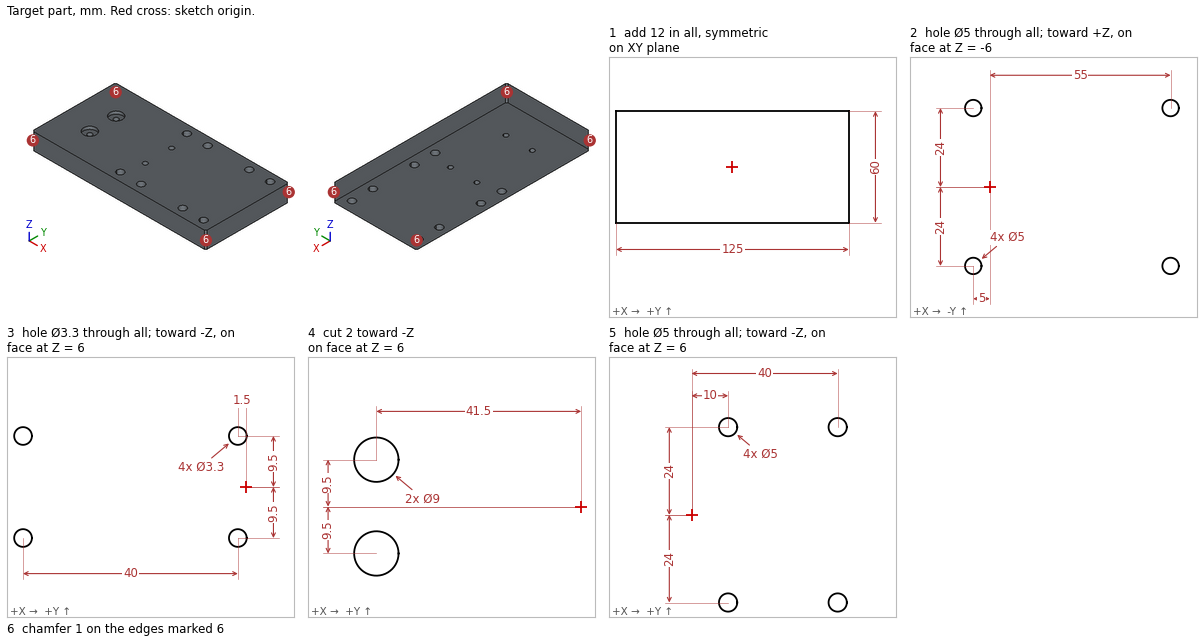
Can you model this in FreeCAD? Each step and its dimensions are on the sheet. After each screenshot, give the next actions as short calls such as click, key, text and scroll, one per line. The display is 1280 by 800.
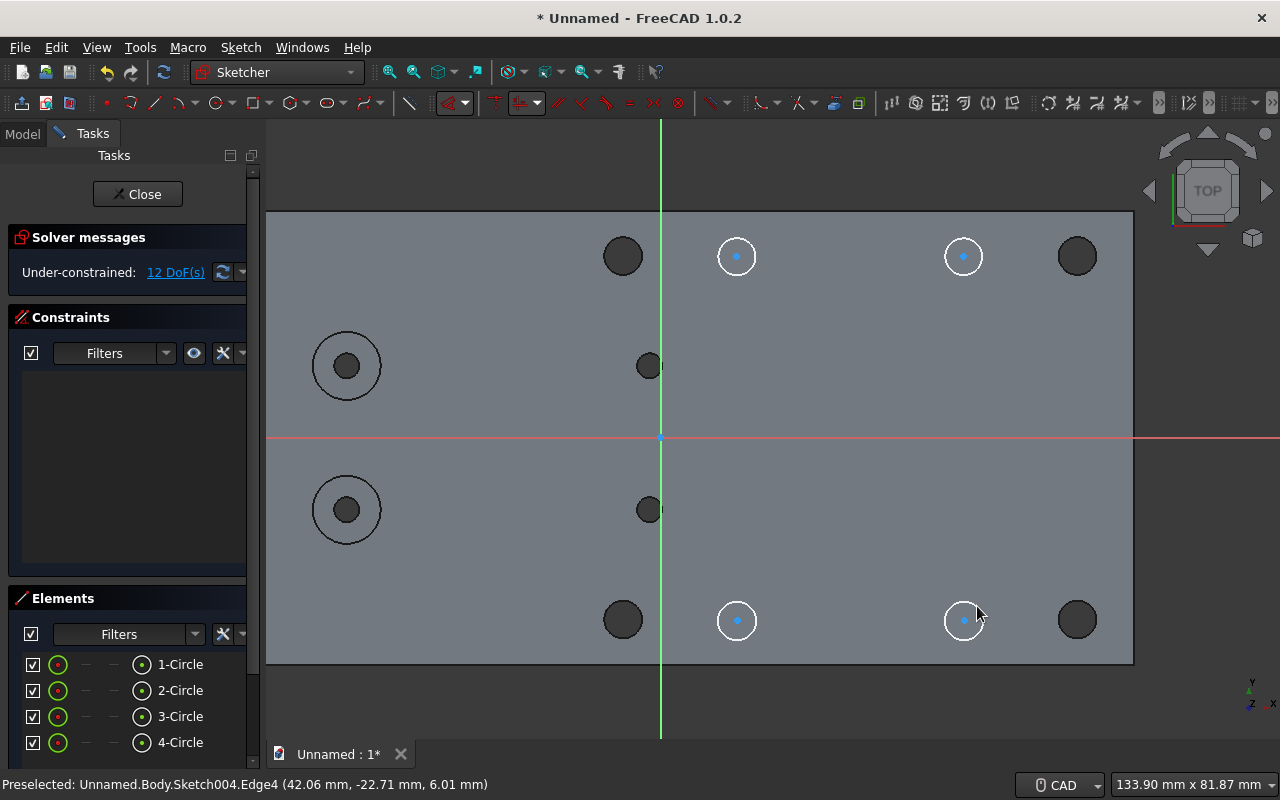
click(750, 244)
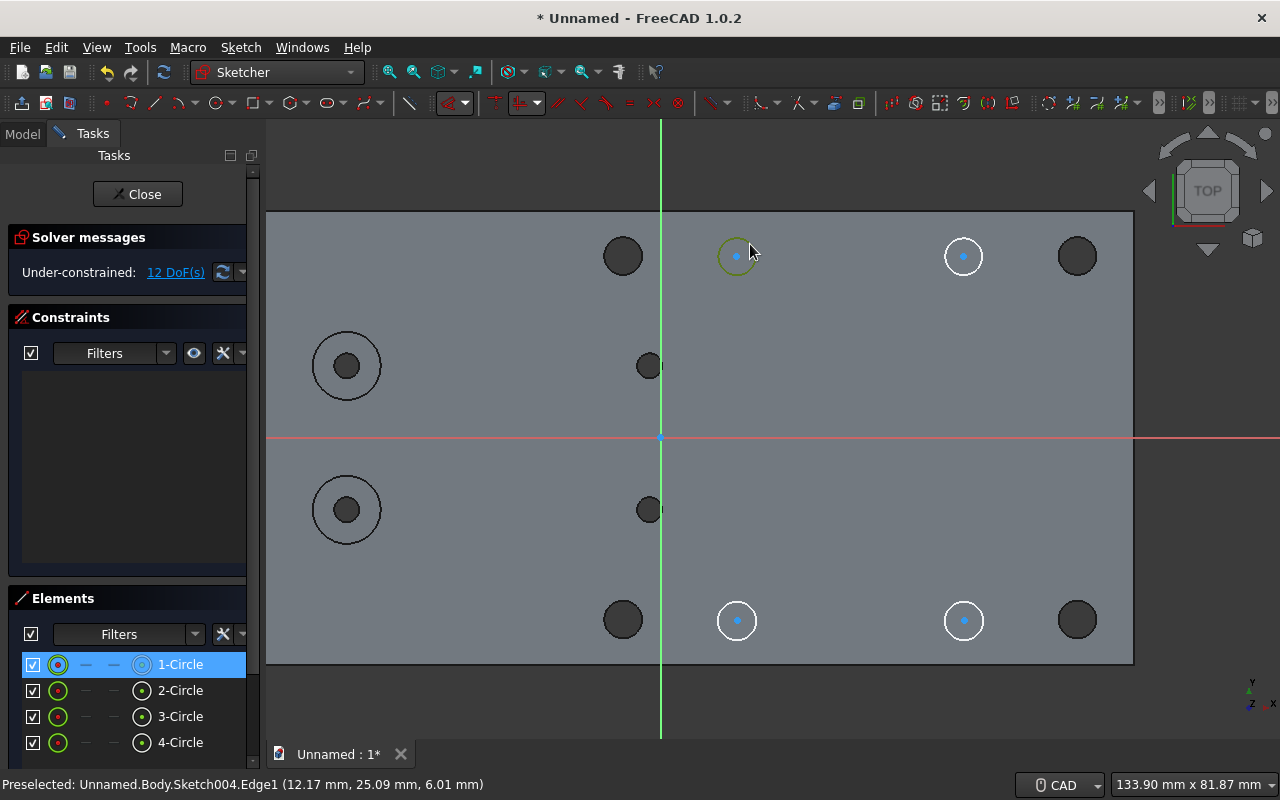
click(977, 244)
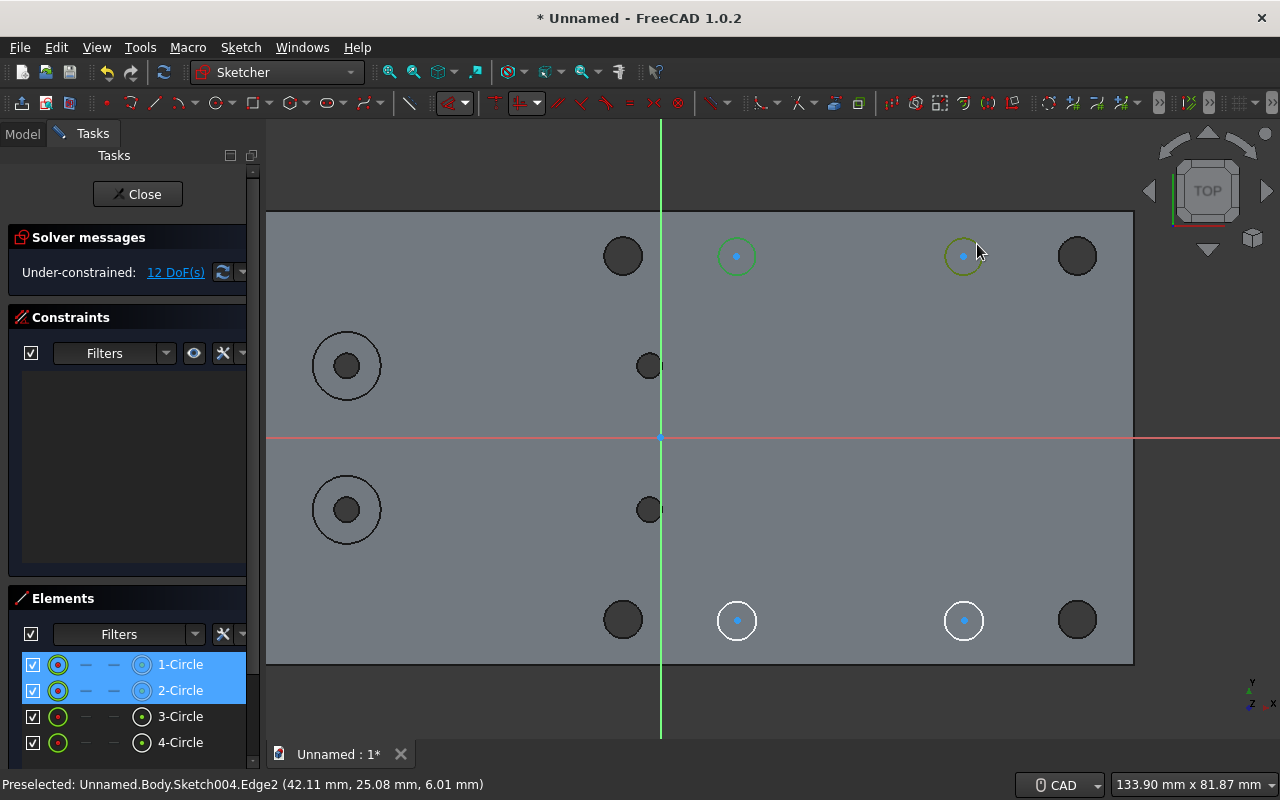
click(750, 607)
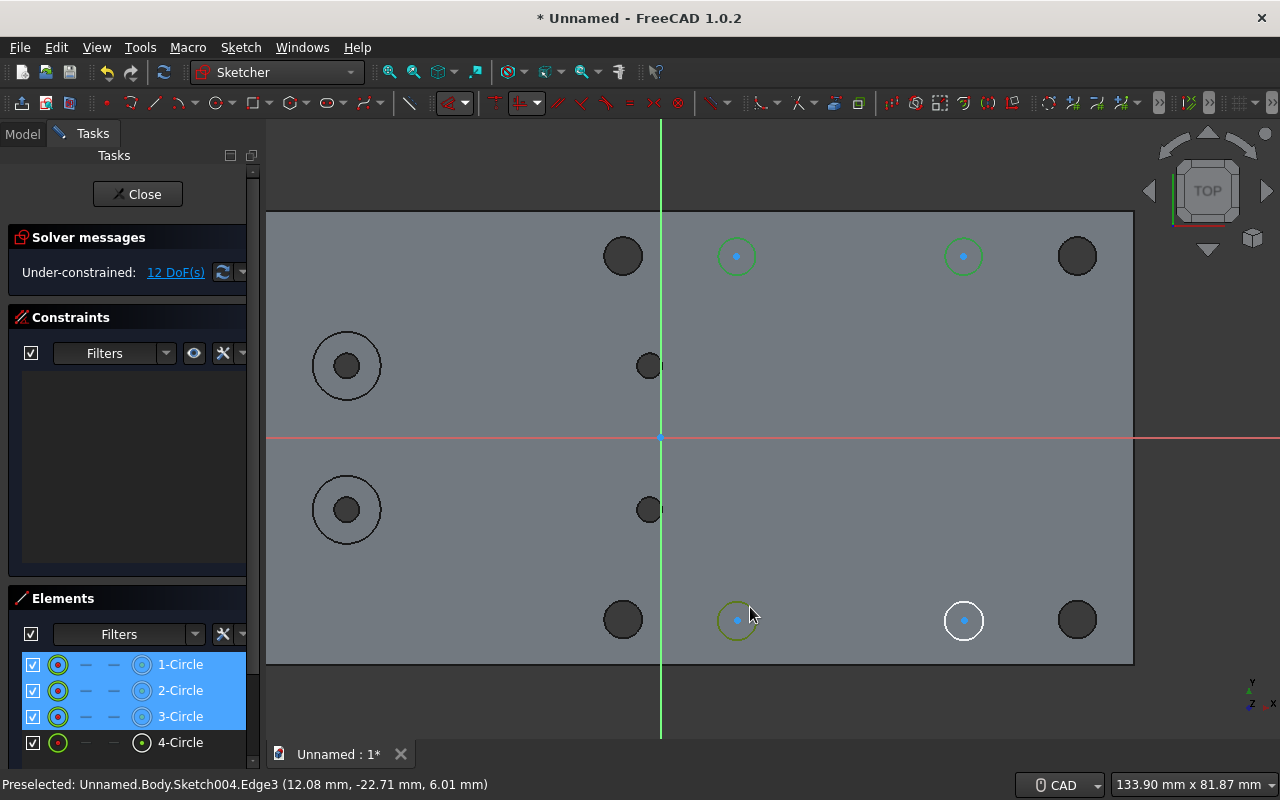
click(977, 607)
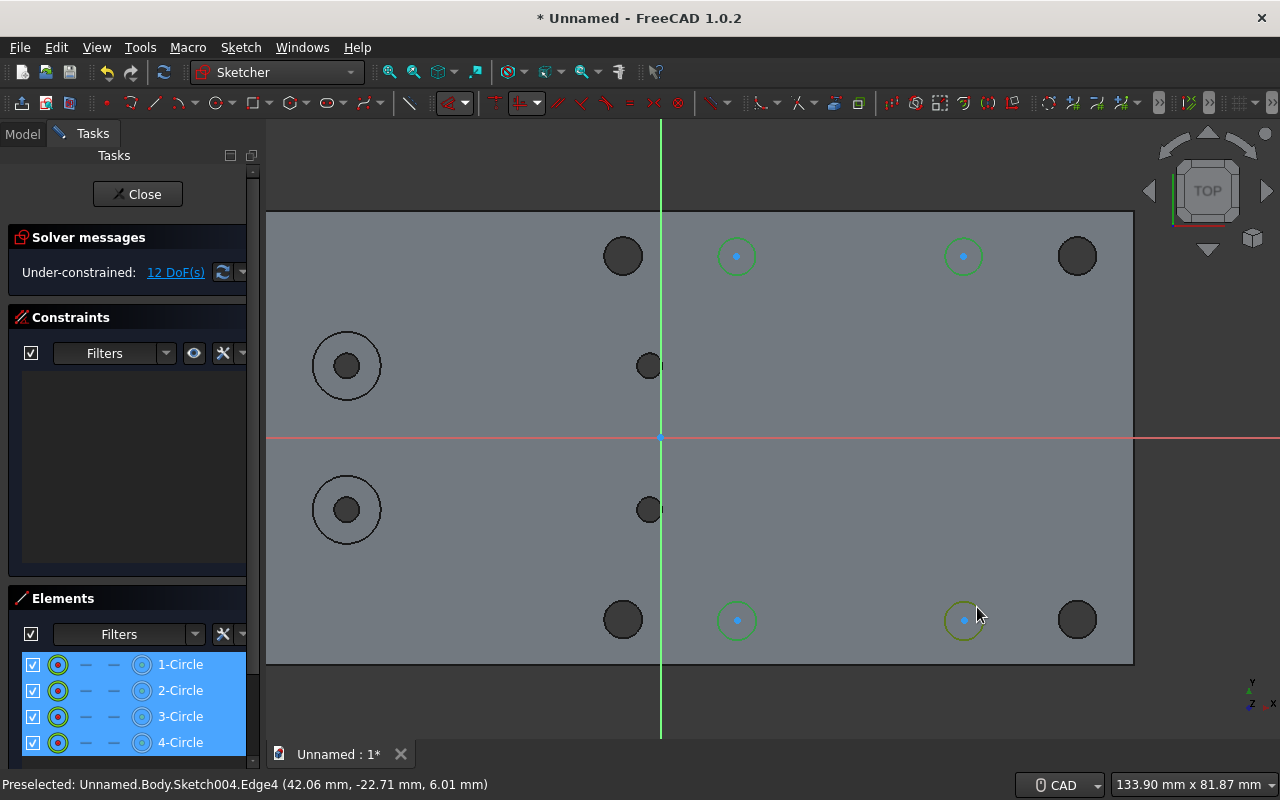
key(e)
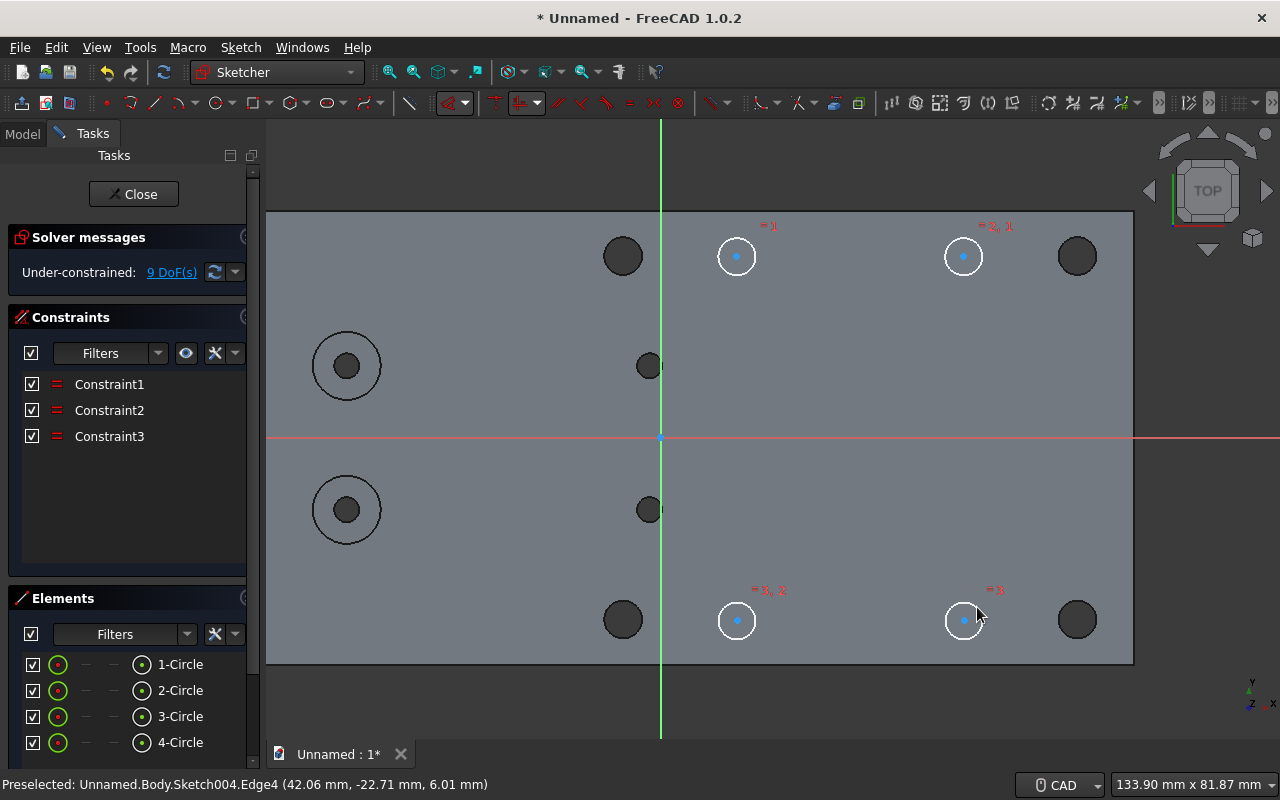
click(737, 257)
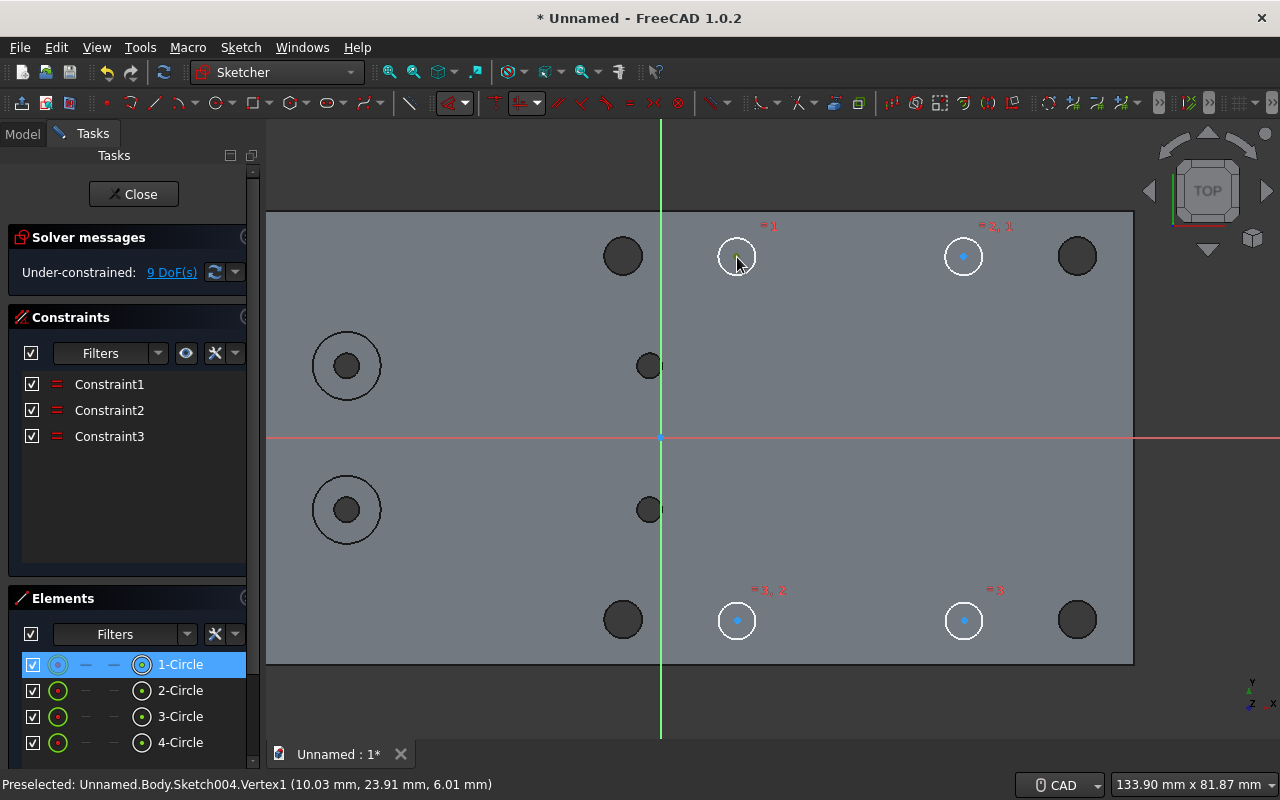
click(964, 257)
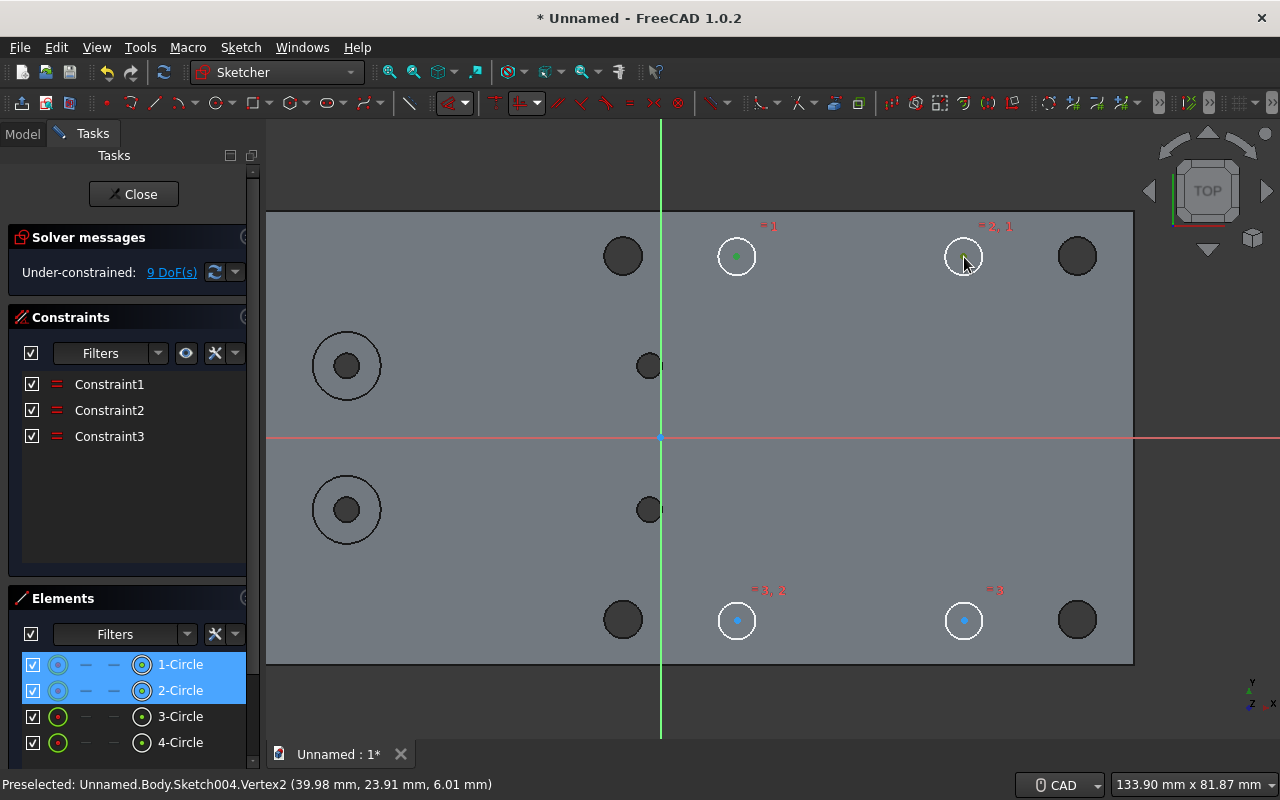
key(h)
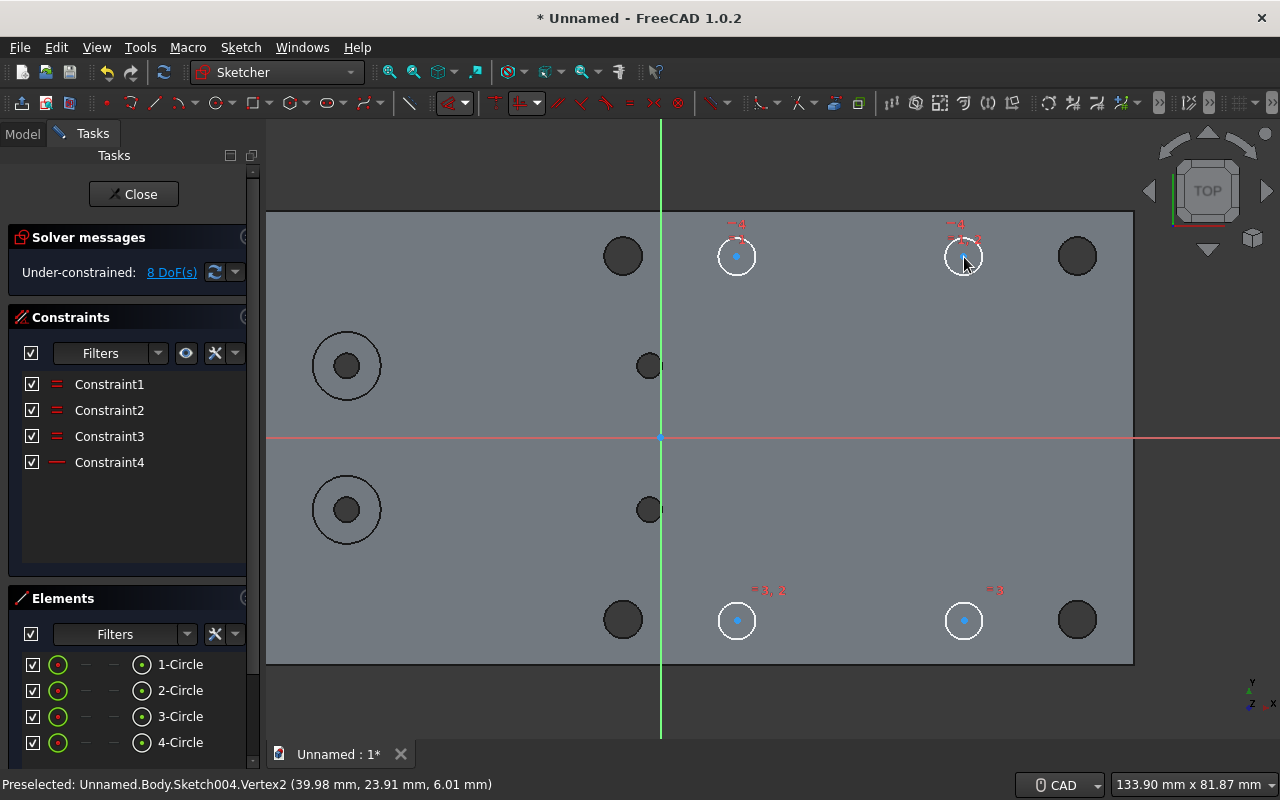
click(737, 257)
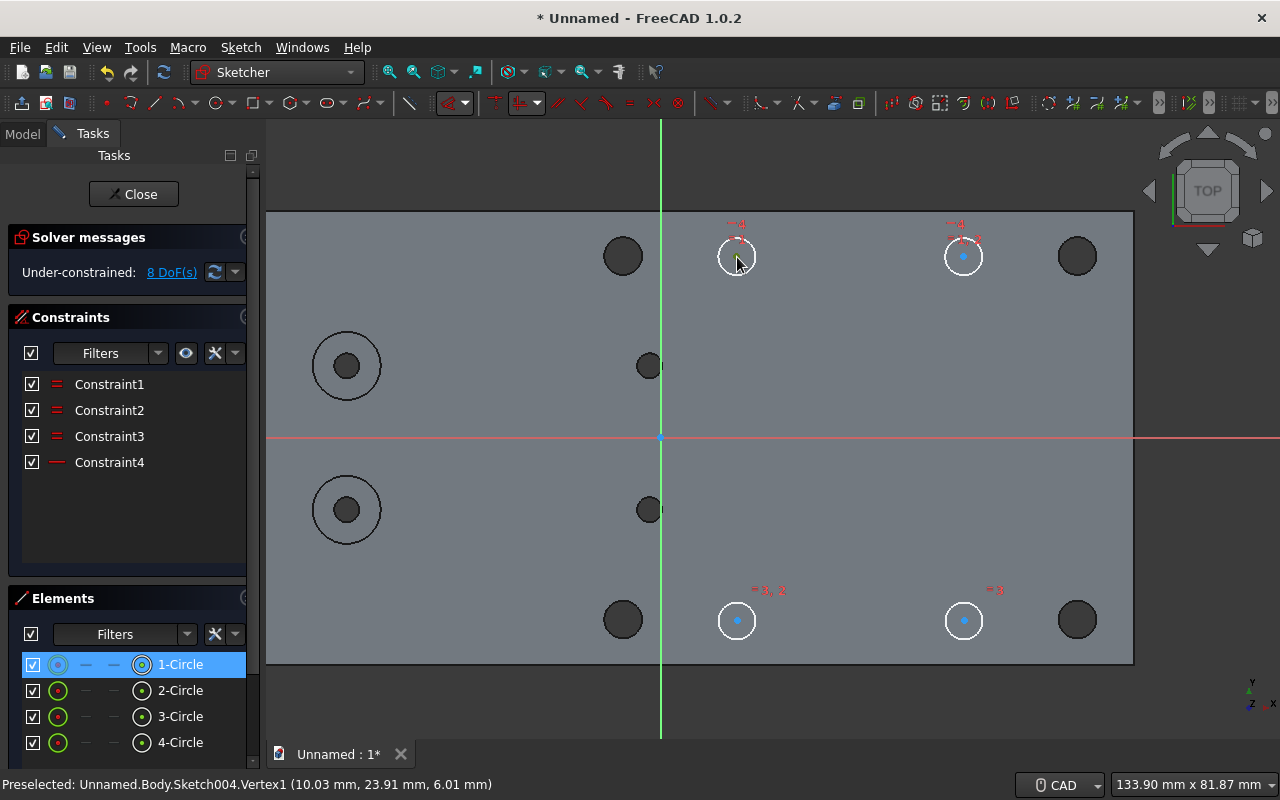
click(737, 621)